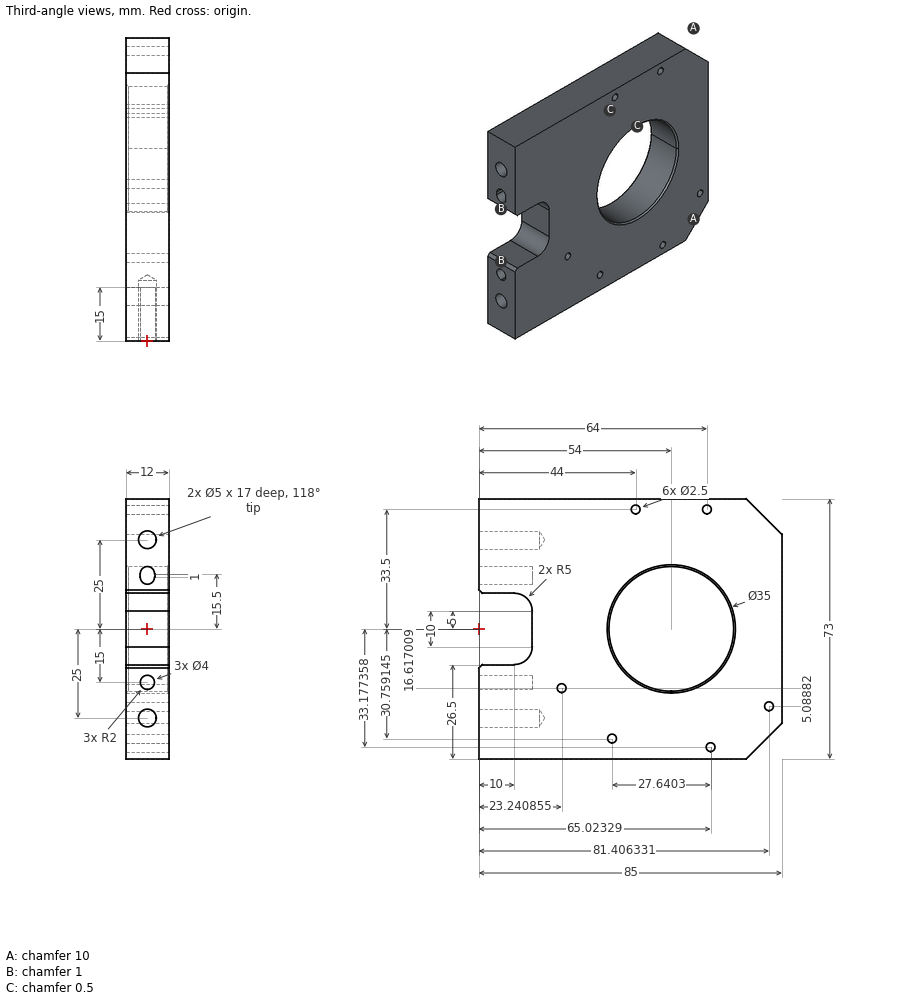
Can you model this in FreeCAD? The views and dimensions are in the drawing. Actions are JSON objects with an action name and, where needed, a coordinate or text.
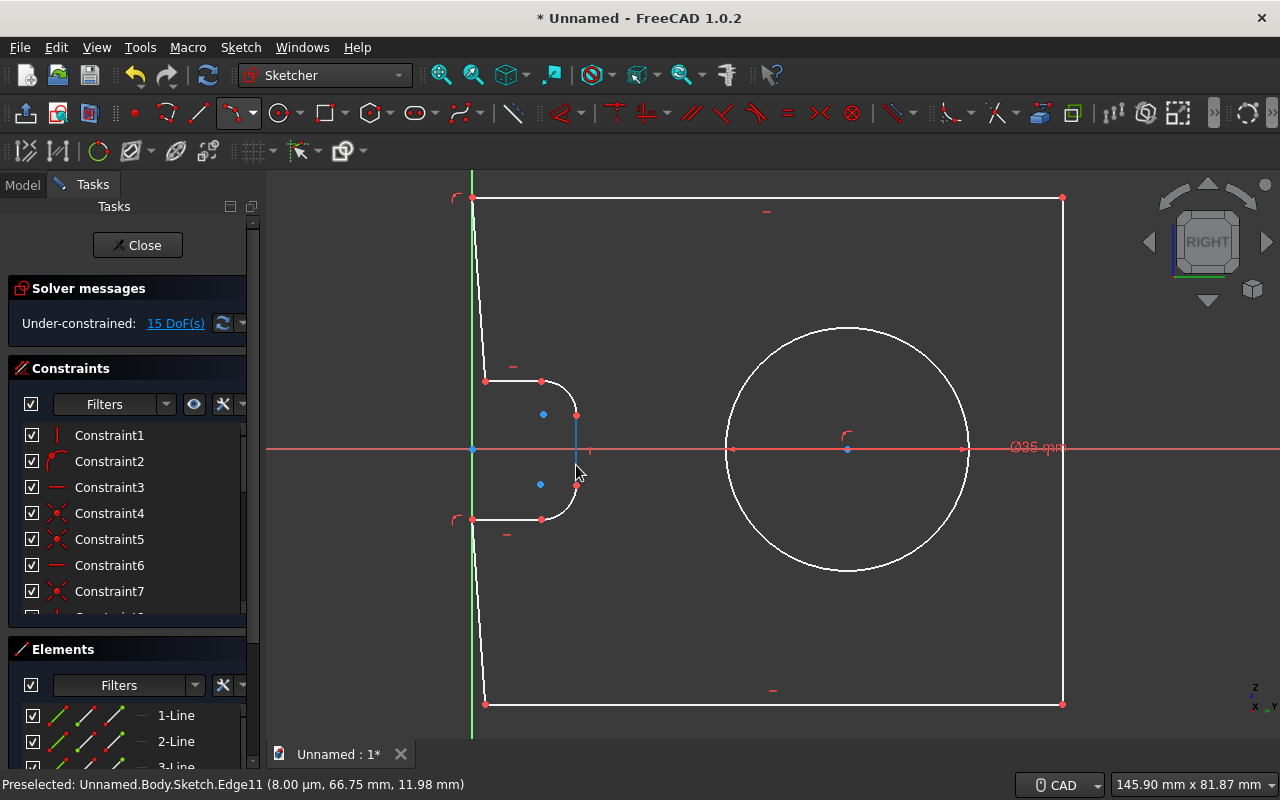
{"action": "left_click", "coordinate": [576, 465]}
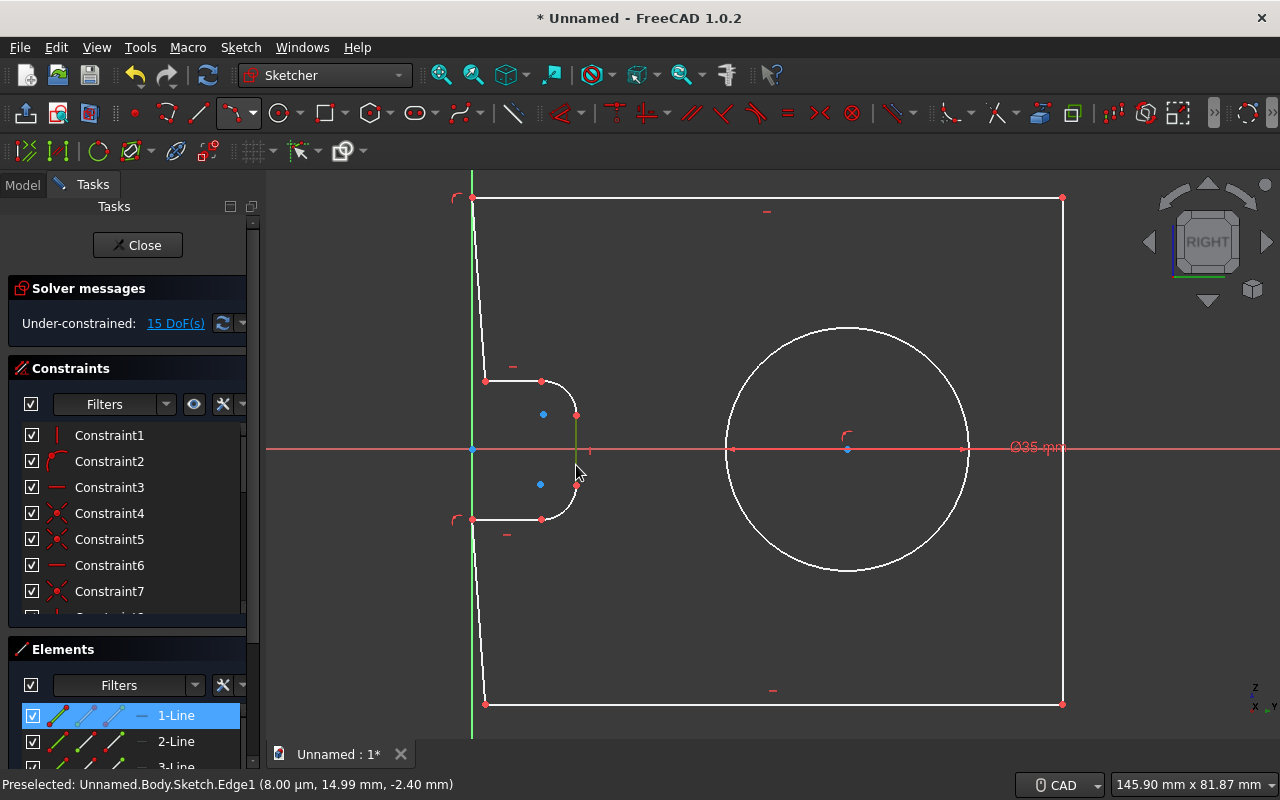
{"action": "left_click", "coordinate": [557, 516]}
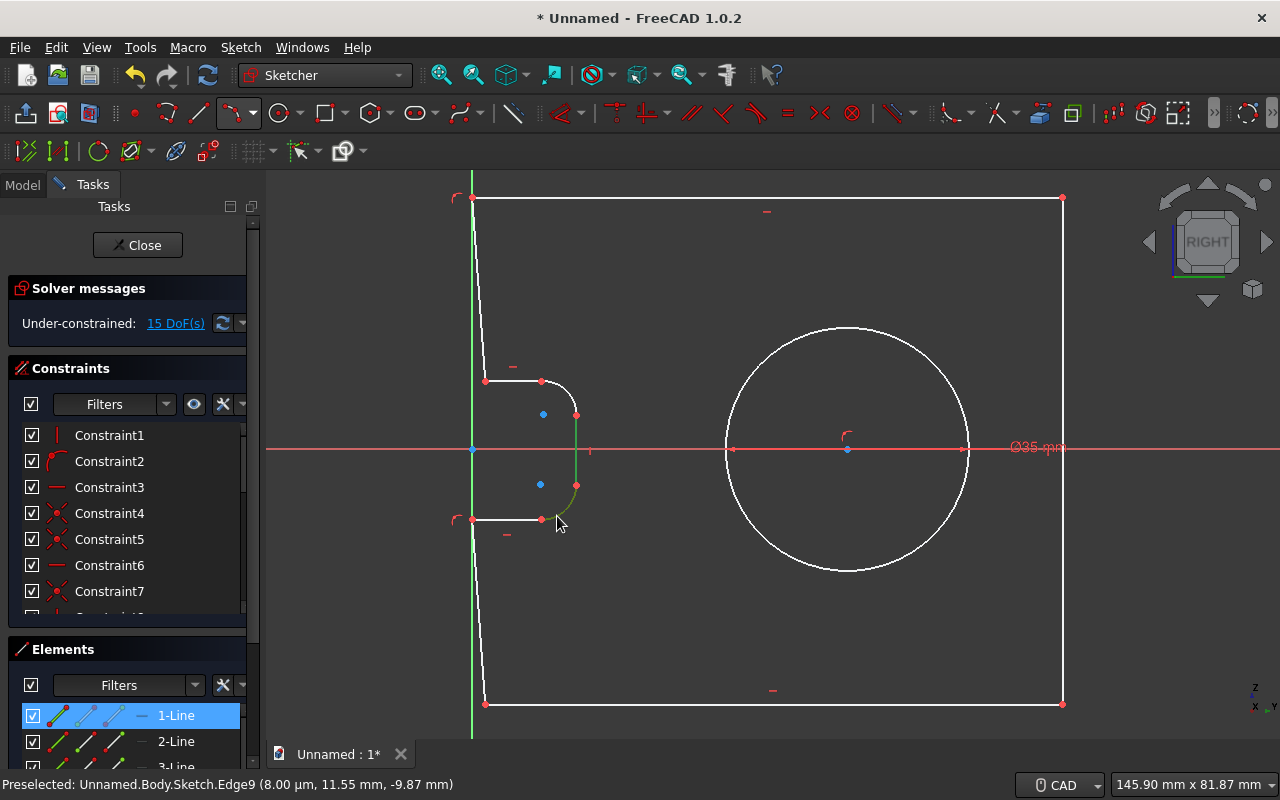
{"action": "left_click", "coordinate": [756, 114]}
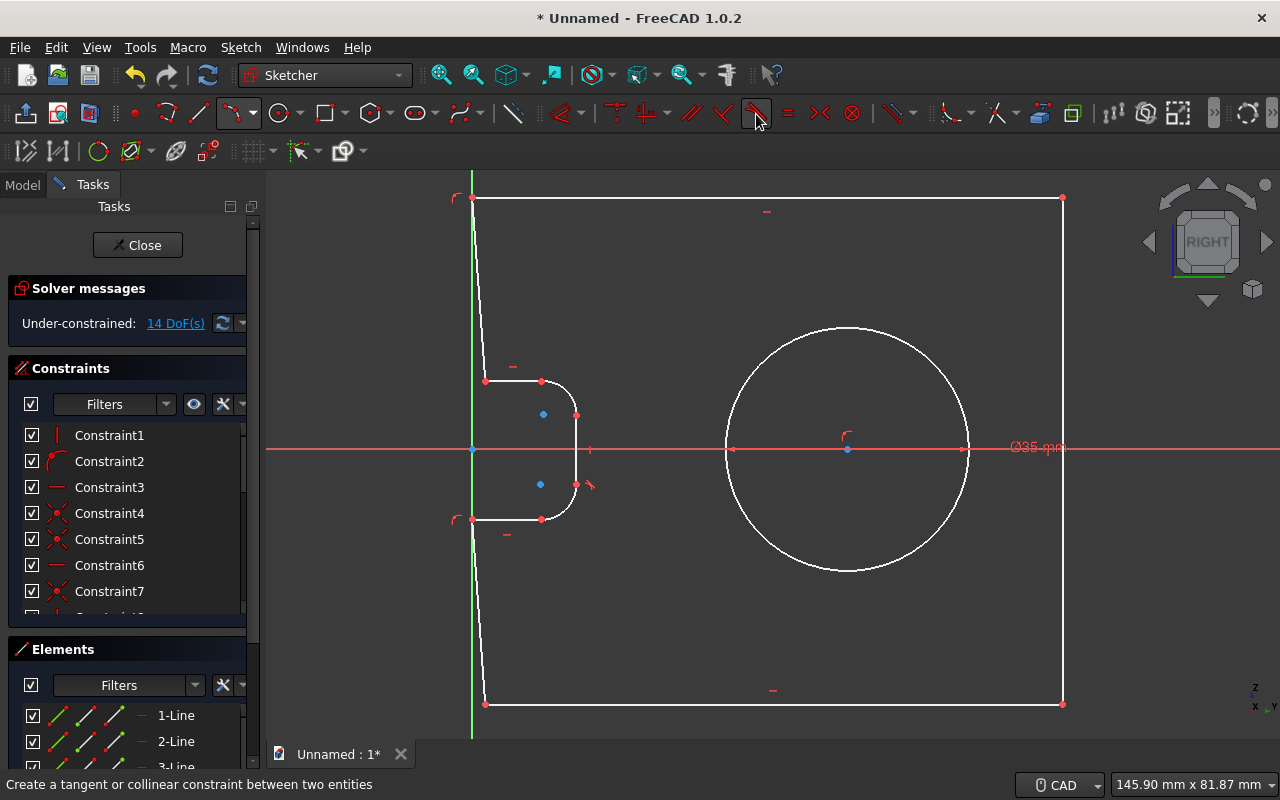
{"action": "left_click", "coordinate": [576, 436]}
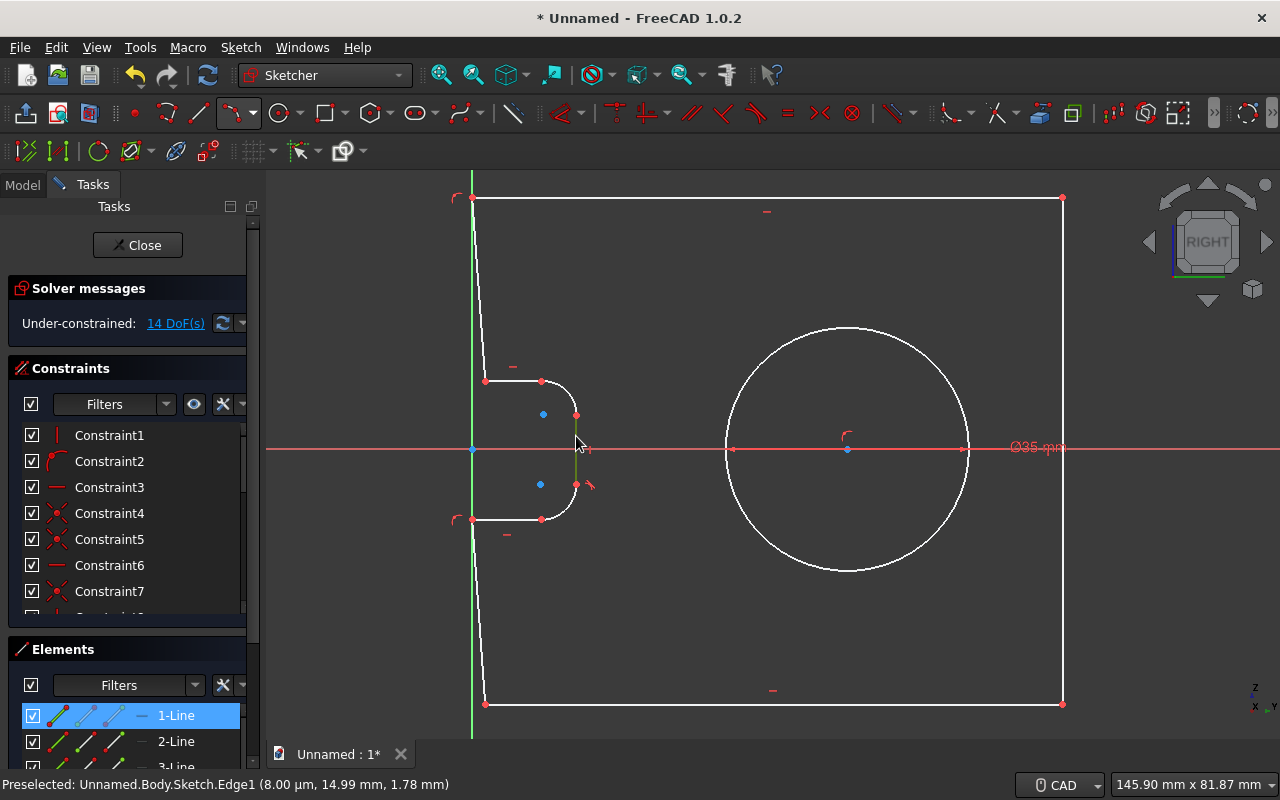
{"action": "left_click", "coordinate": [573, 400]}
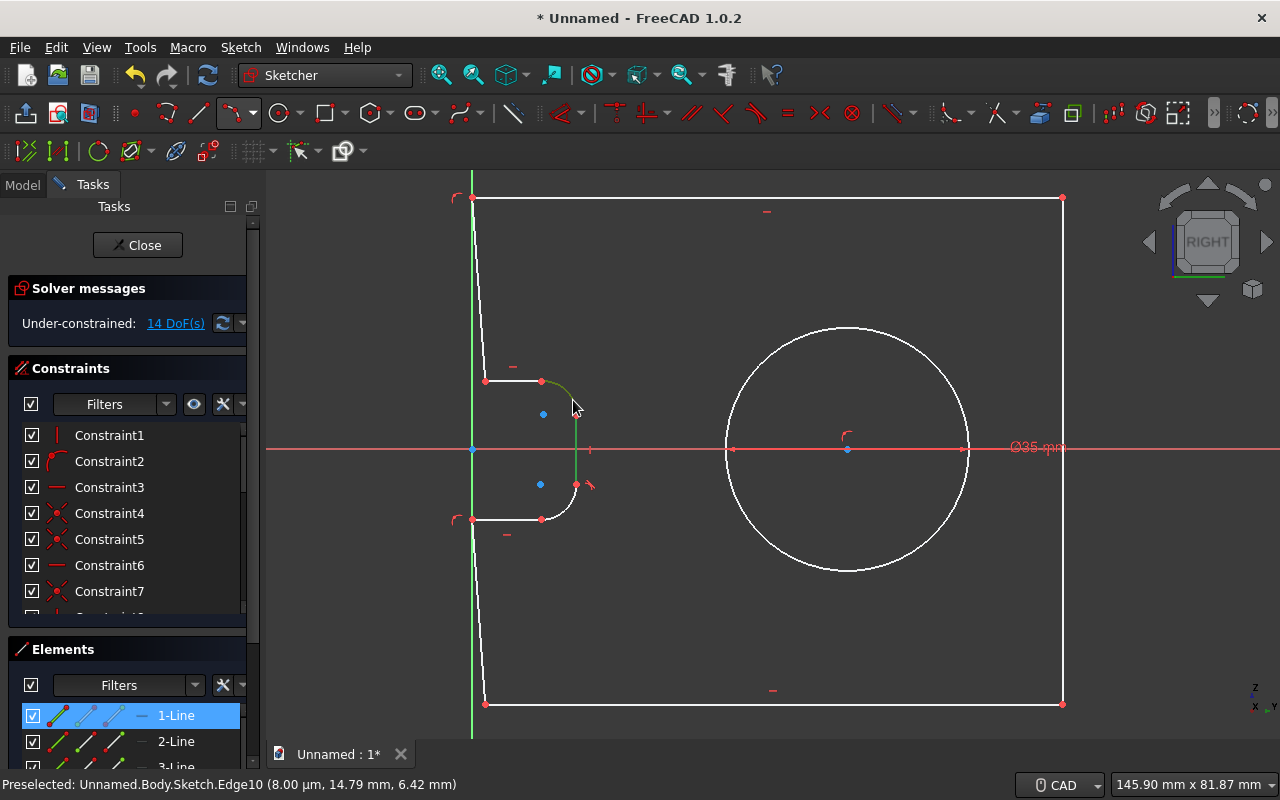
{"action": "left_click", "coordinate": [756, 114]}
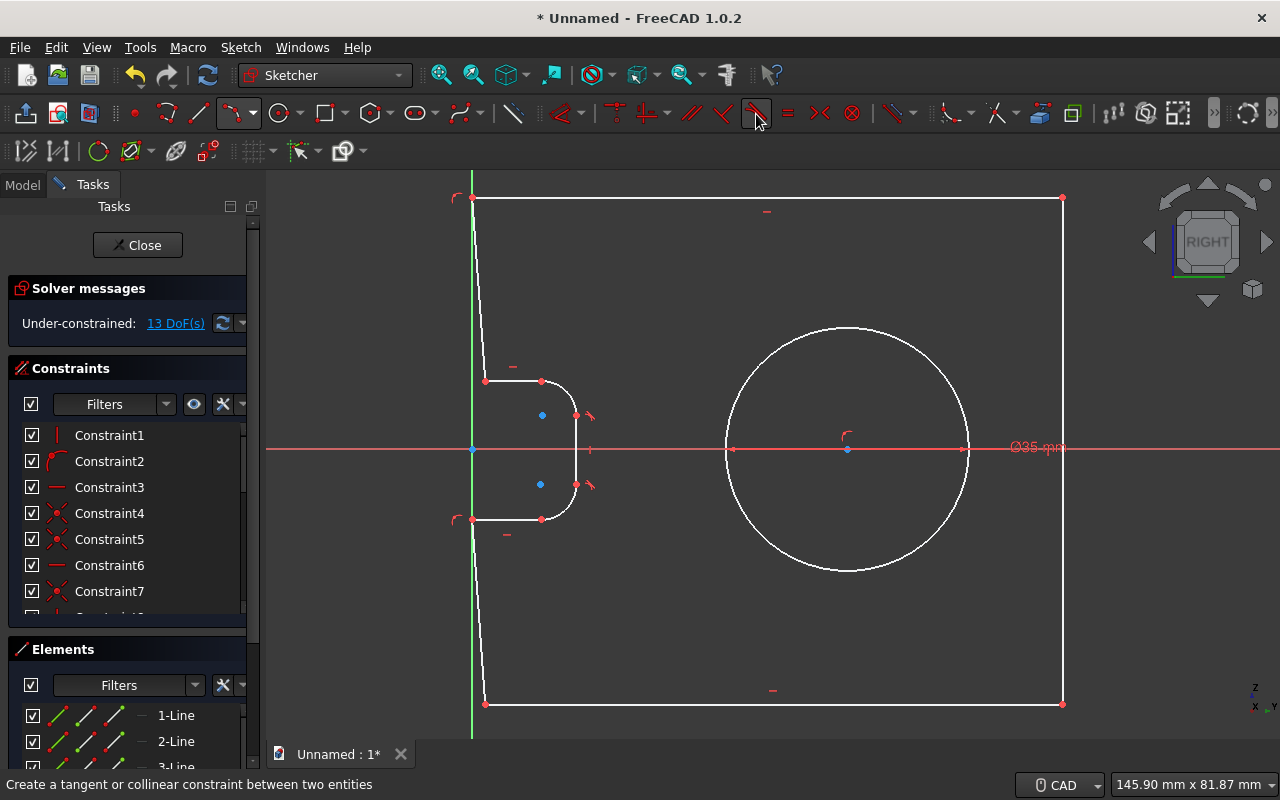
{"action": "left_click", "coordinate": [521, 520]}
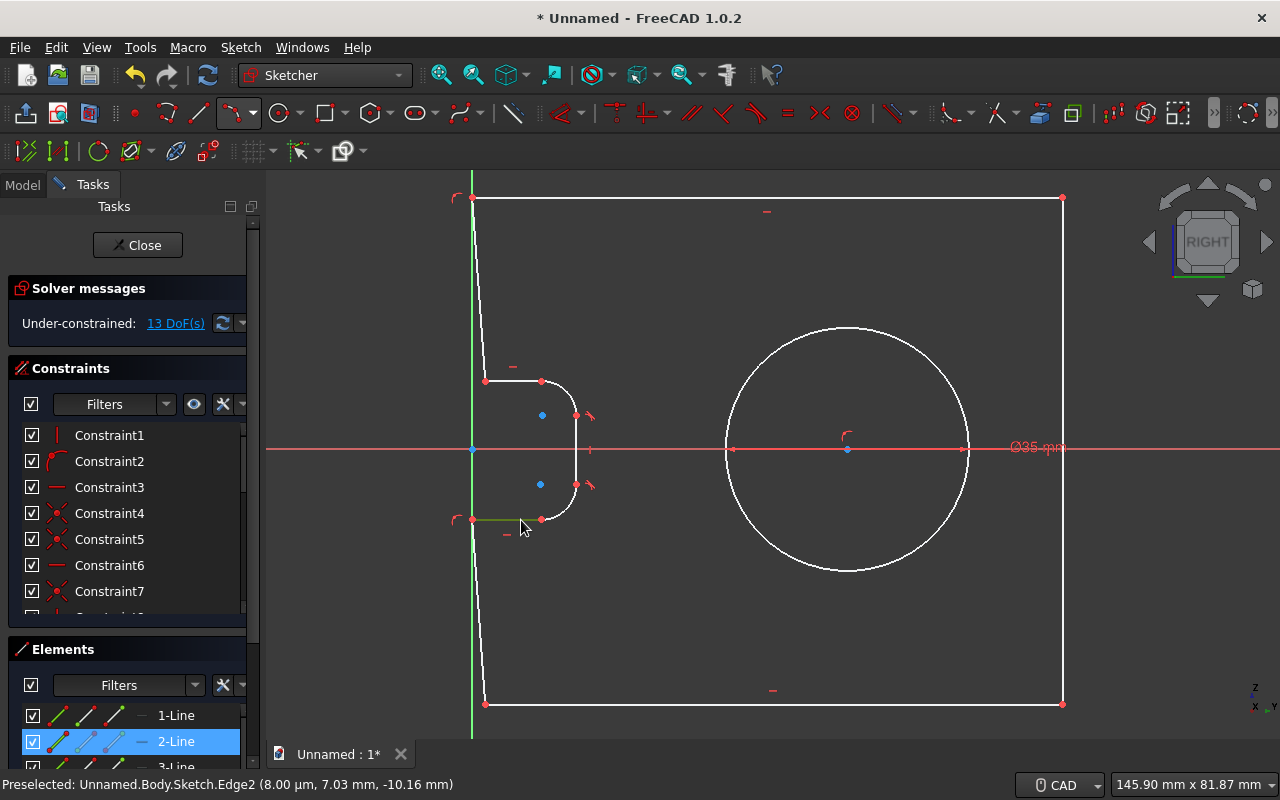
{"action": "left_click", "coordinate": [558, 516]}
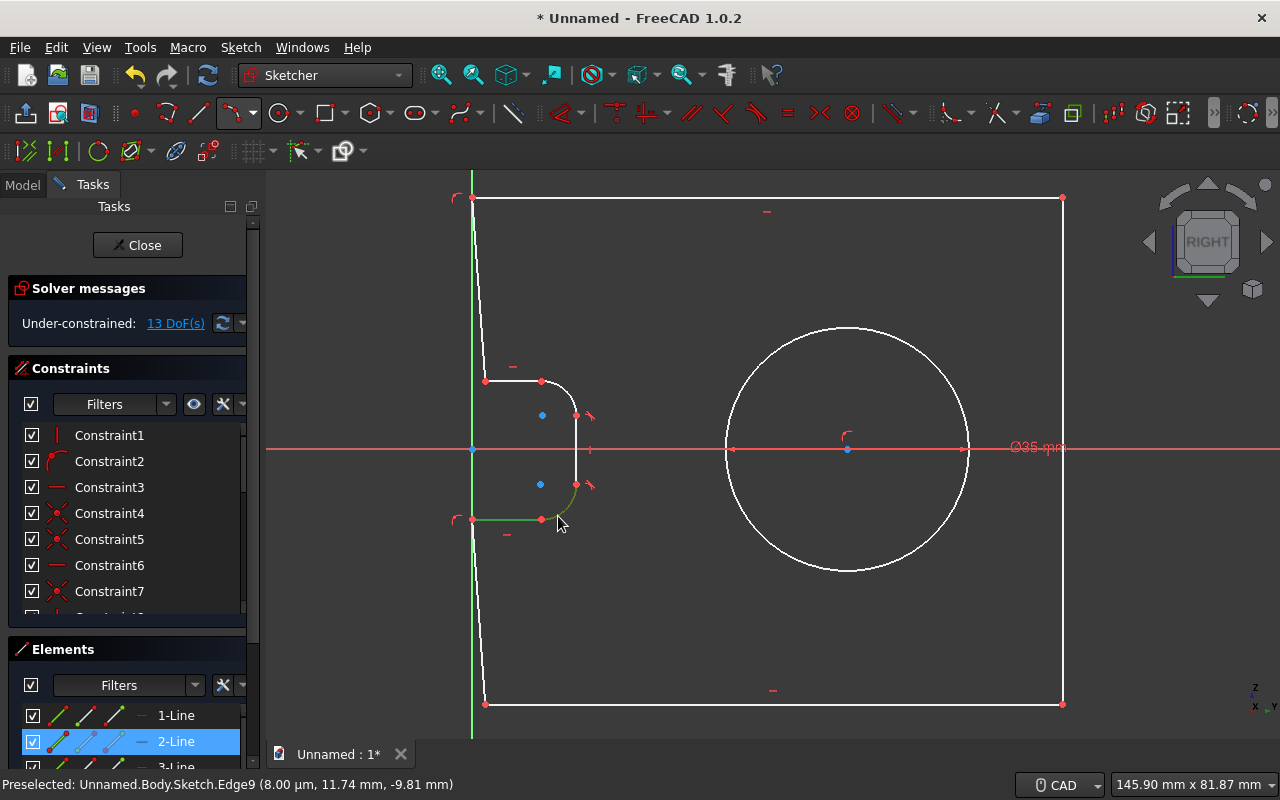
{"action": "left_click", "coordinate": [756, 114]}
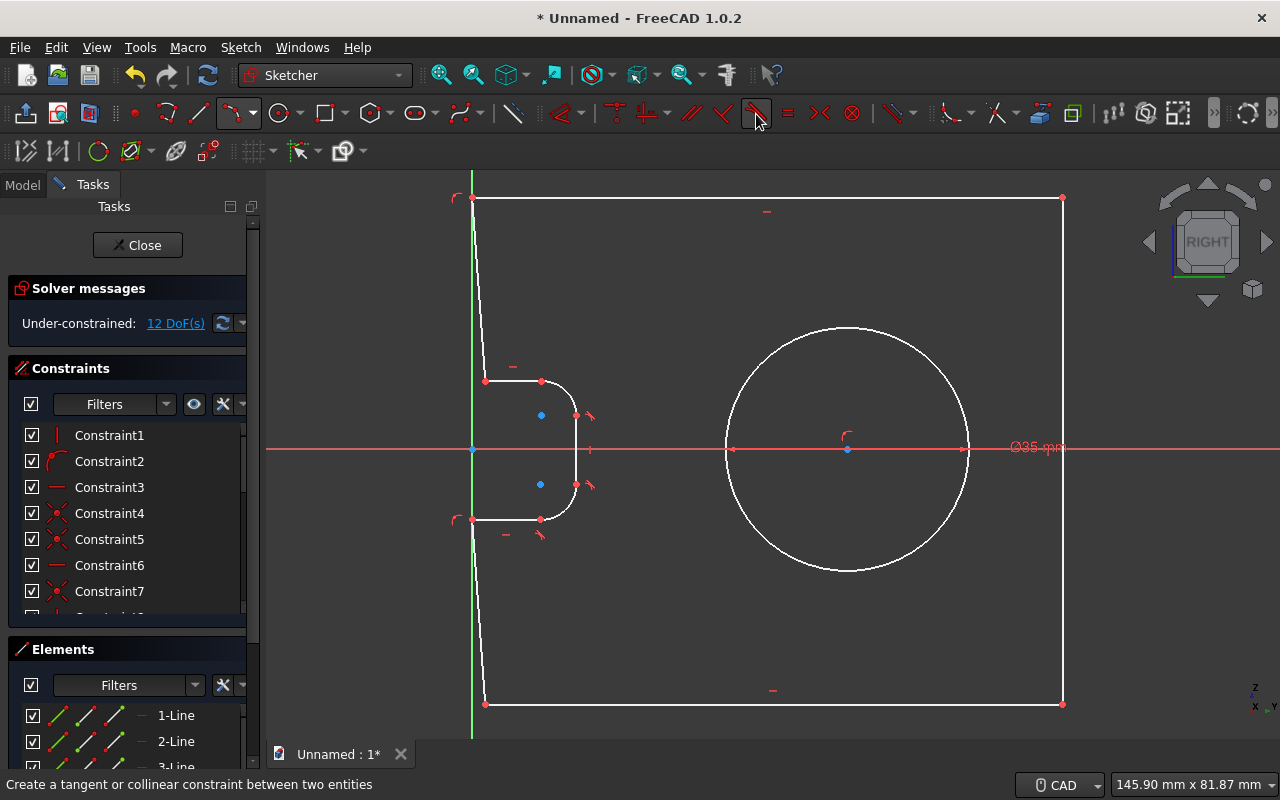
{"action": "left_click", "coordinate": [502, 381]}